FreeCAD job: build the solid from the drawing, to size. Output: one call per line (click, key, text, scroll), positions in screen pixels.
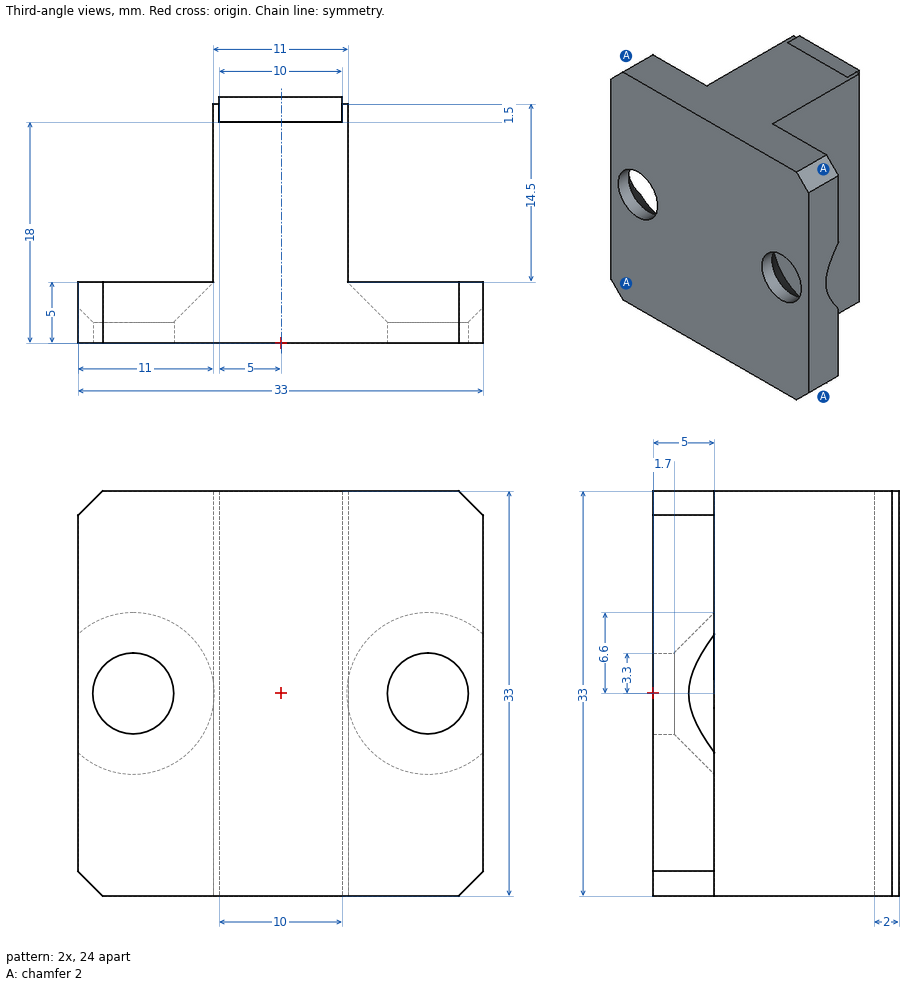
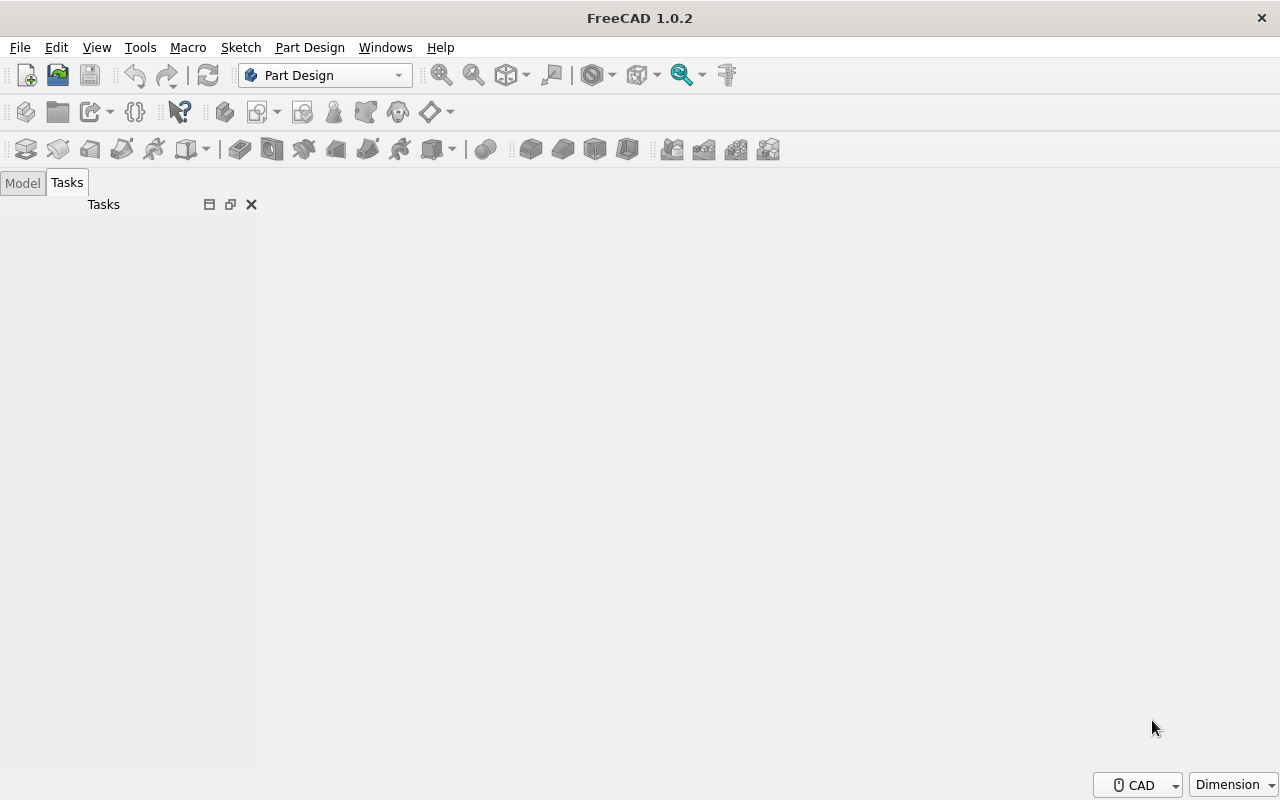
click(26, 76)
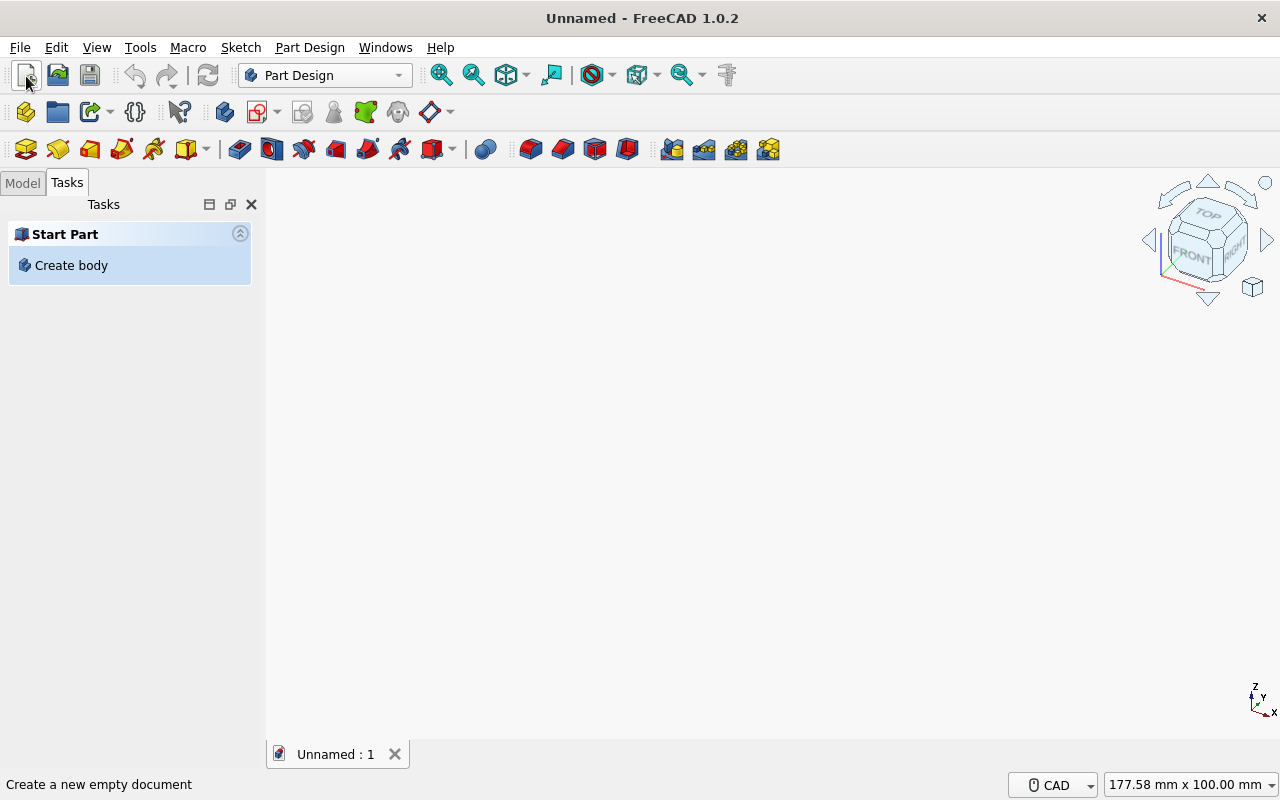
click(258, 112)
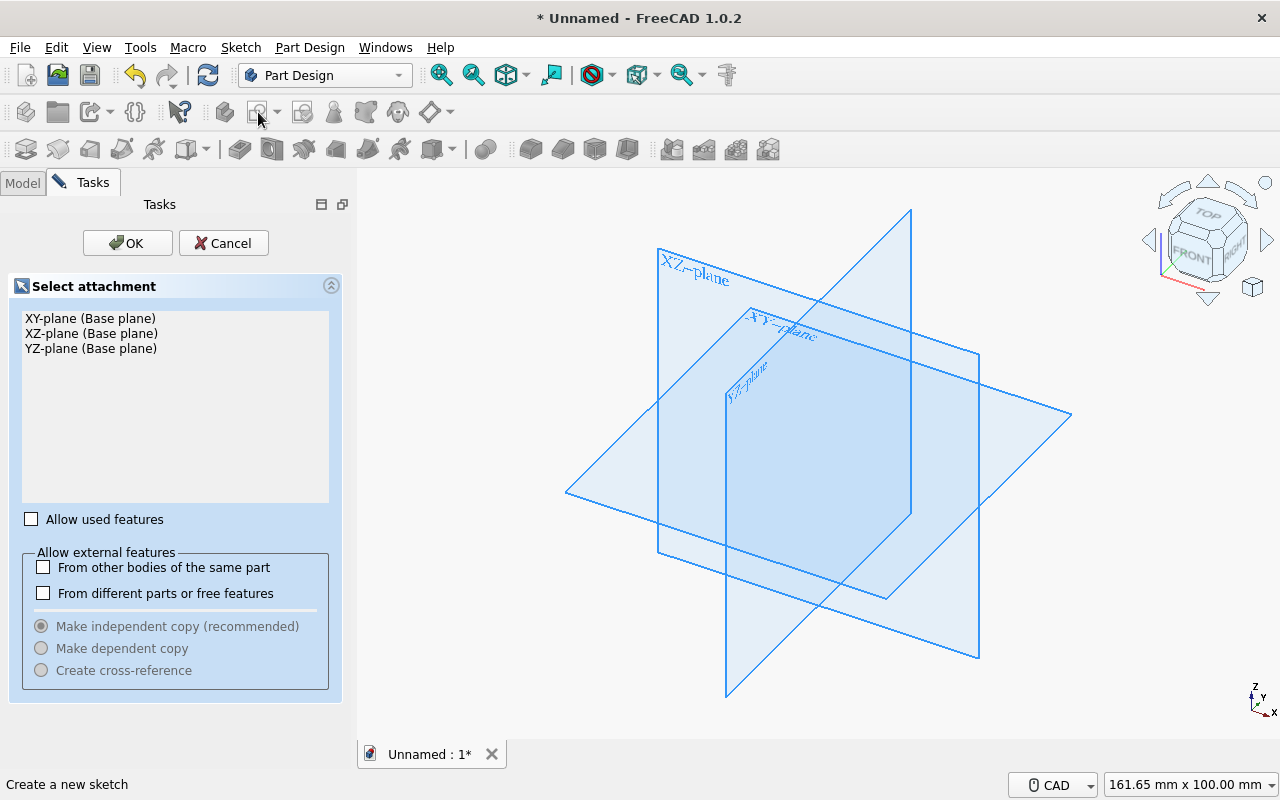
click(82, 318)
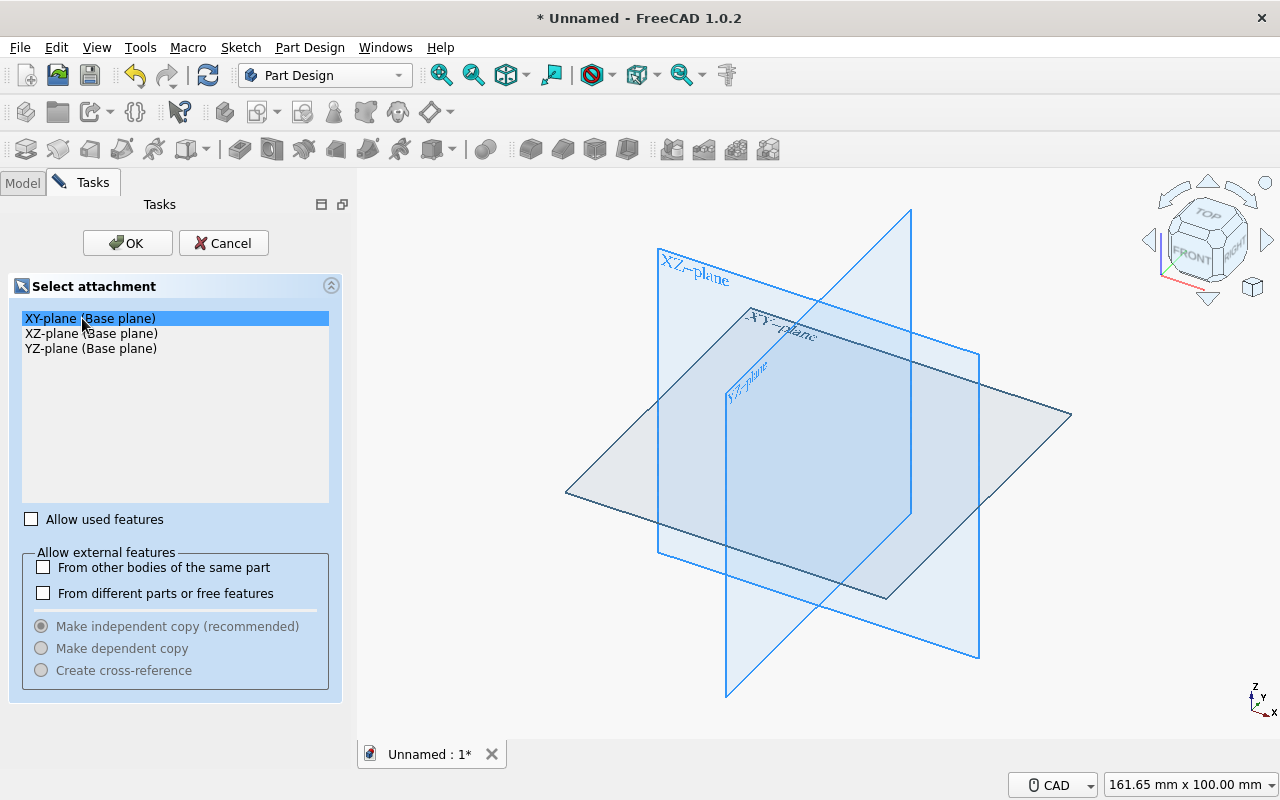
click(128, 243)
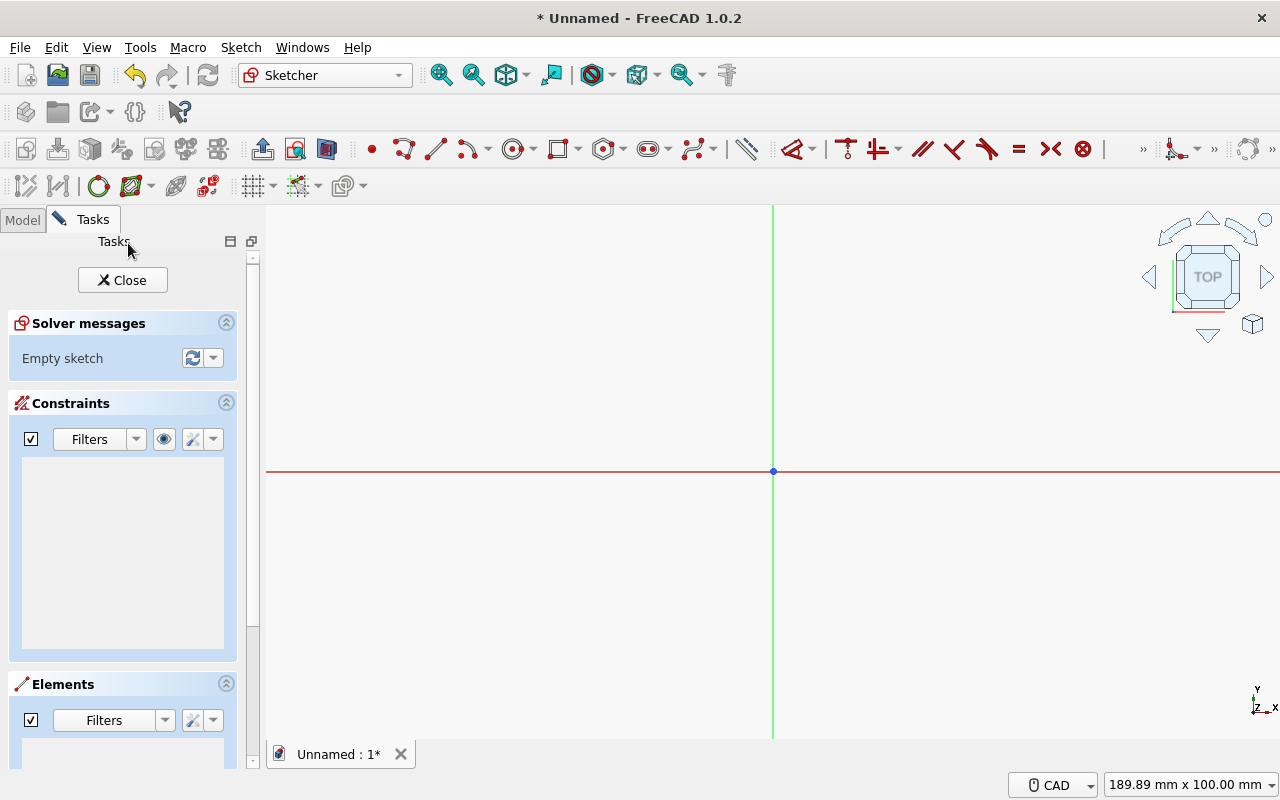
scroll(803, 397, up, 6)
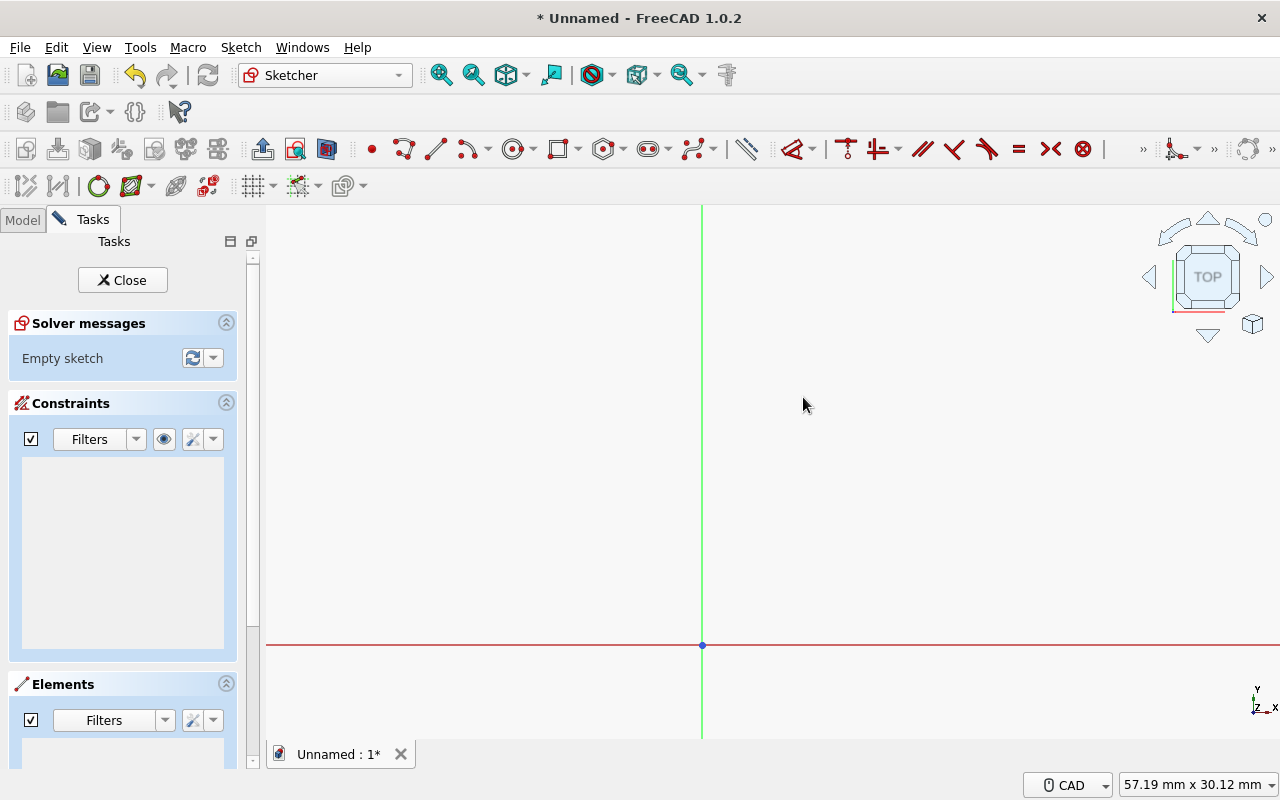
click(404, 150)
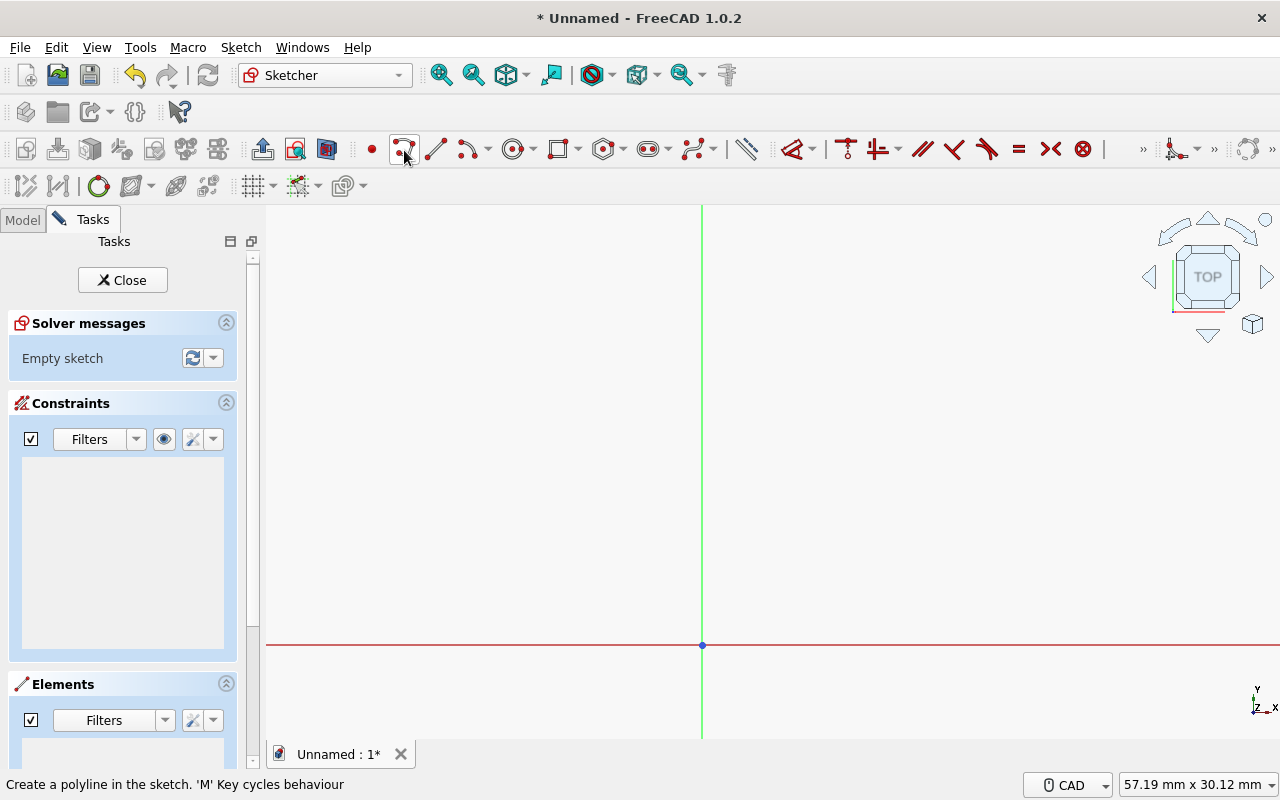
click(800, 557)
click(800, 299)
click(605, 299)
click(605, 557)
click(410, 557)
click(410, 645)
click(995, 636)
click(995, 557)
click(800, 558)
key(Escape)
key(Escape)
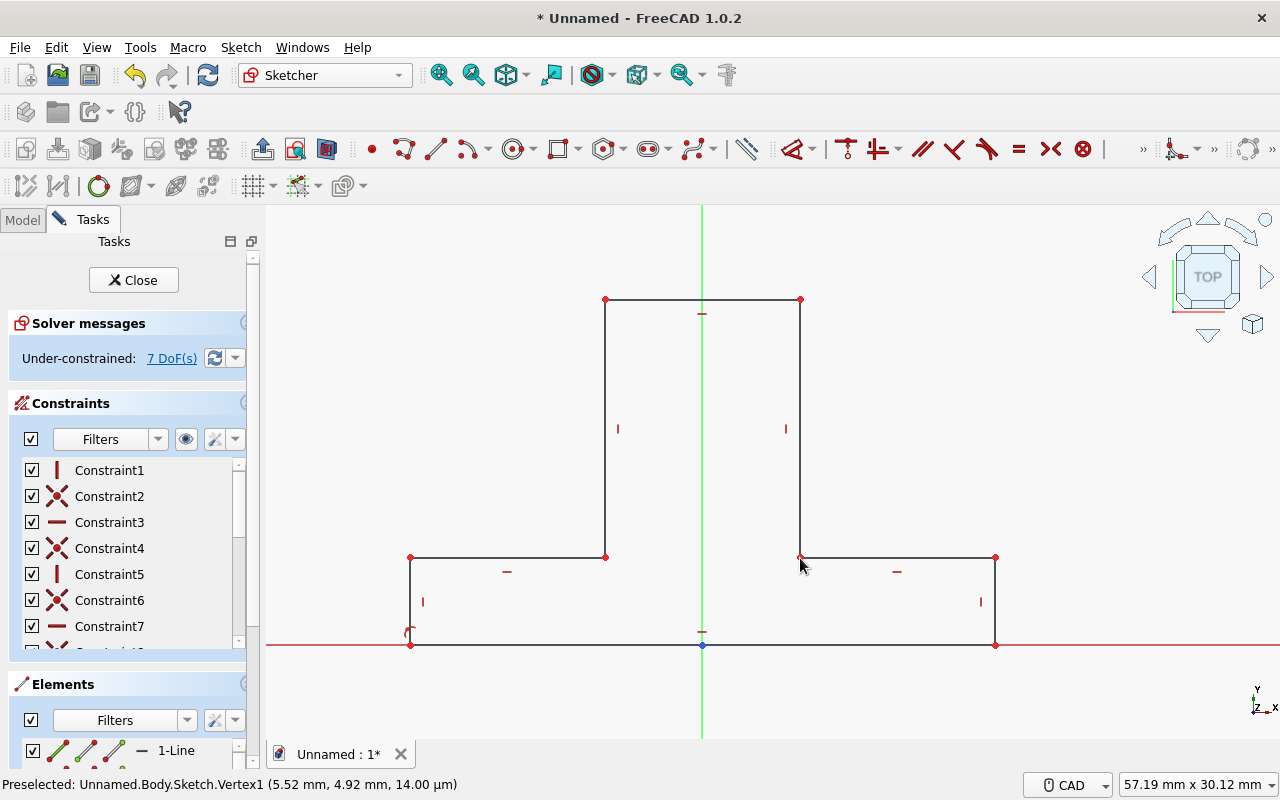
click(800, 558)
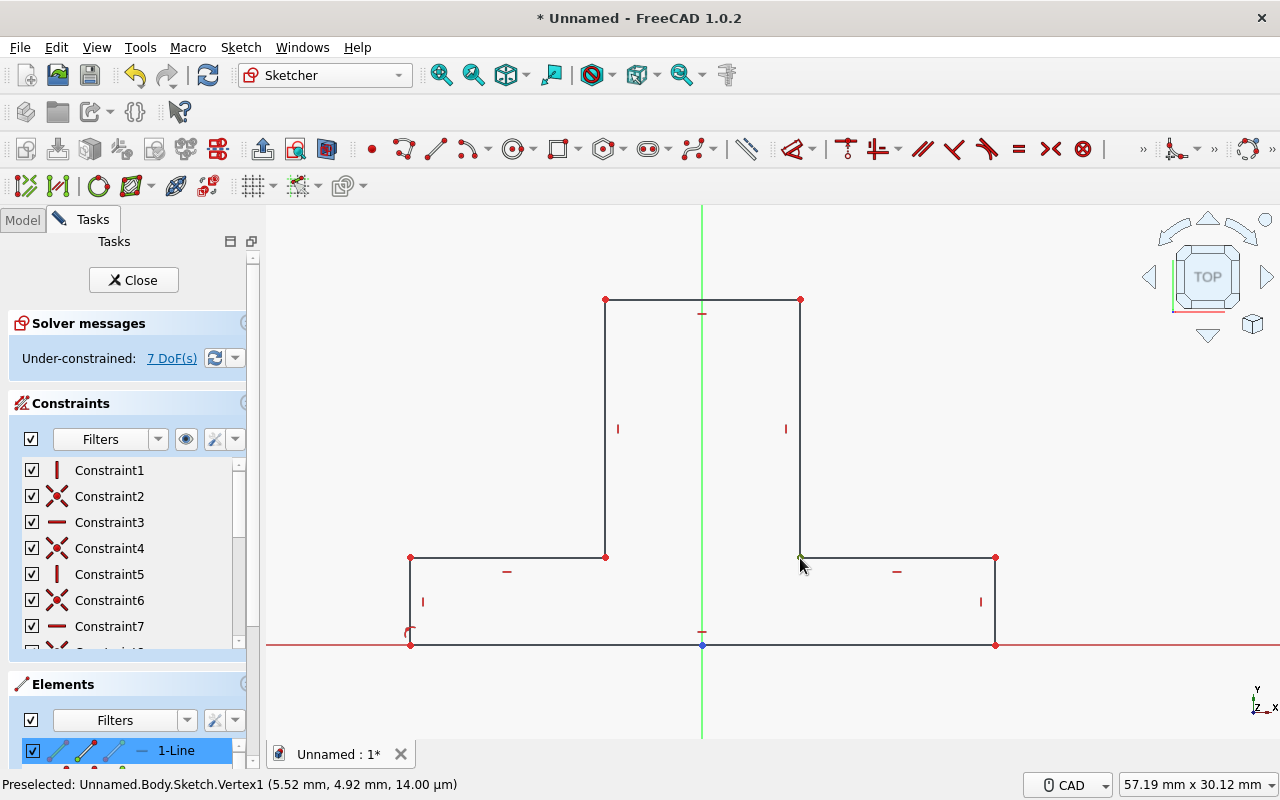
click(605, 558)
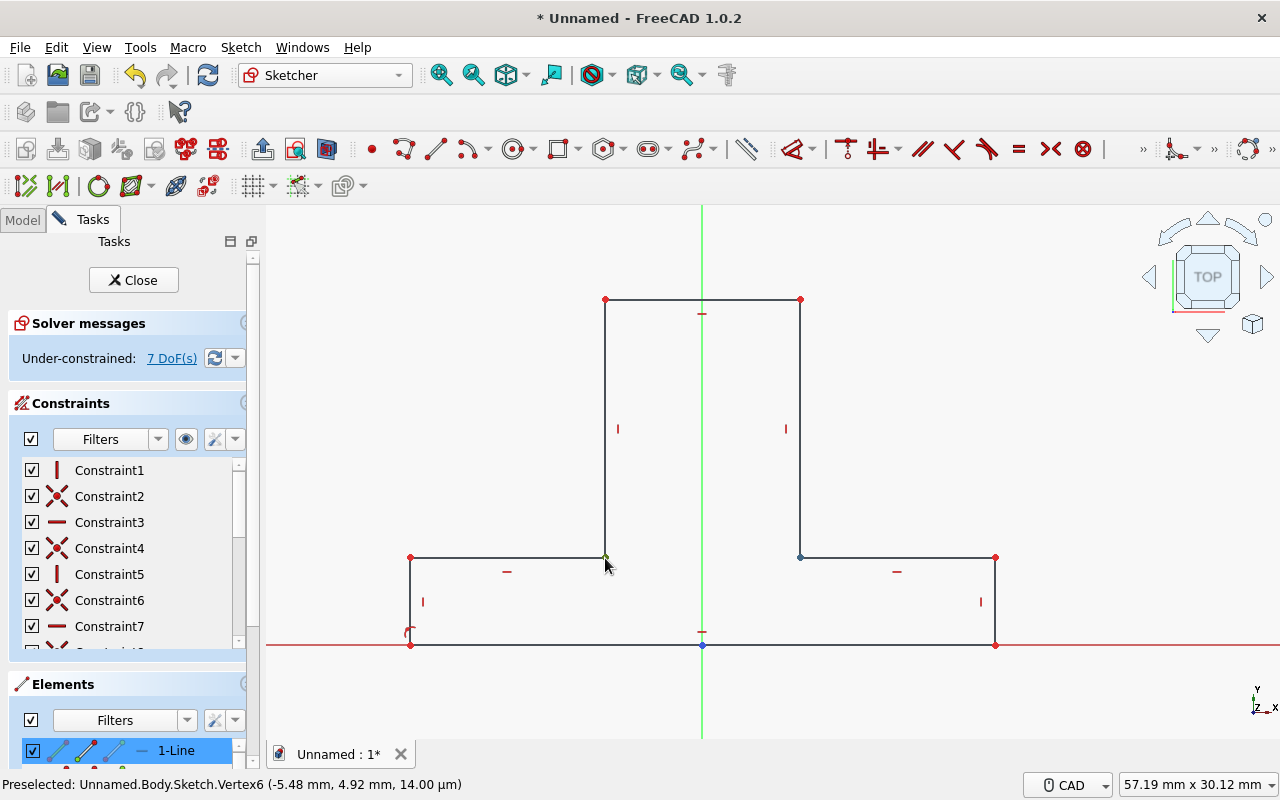
click(702, 677)